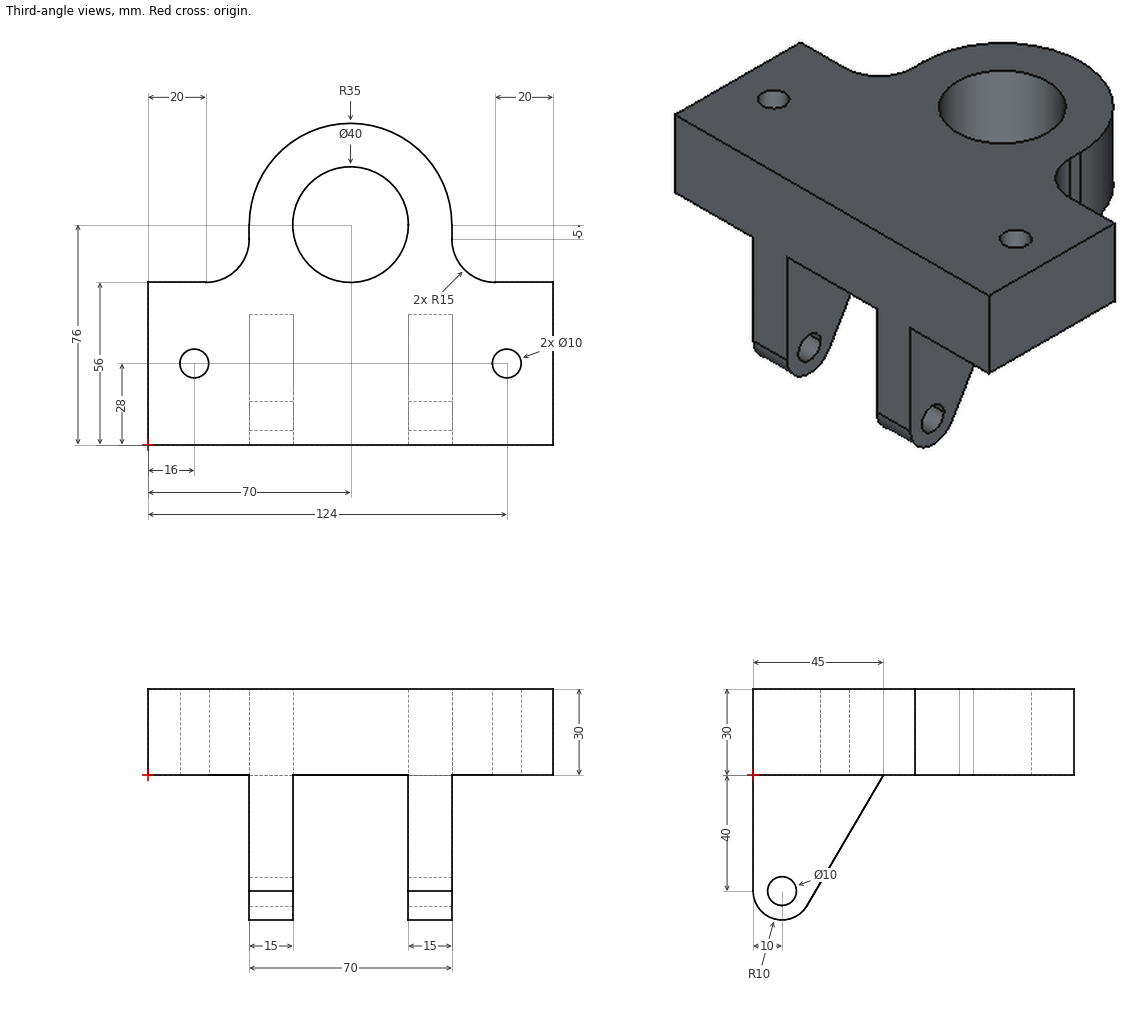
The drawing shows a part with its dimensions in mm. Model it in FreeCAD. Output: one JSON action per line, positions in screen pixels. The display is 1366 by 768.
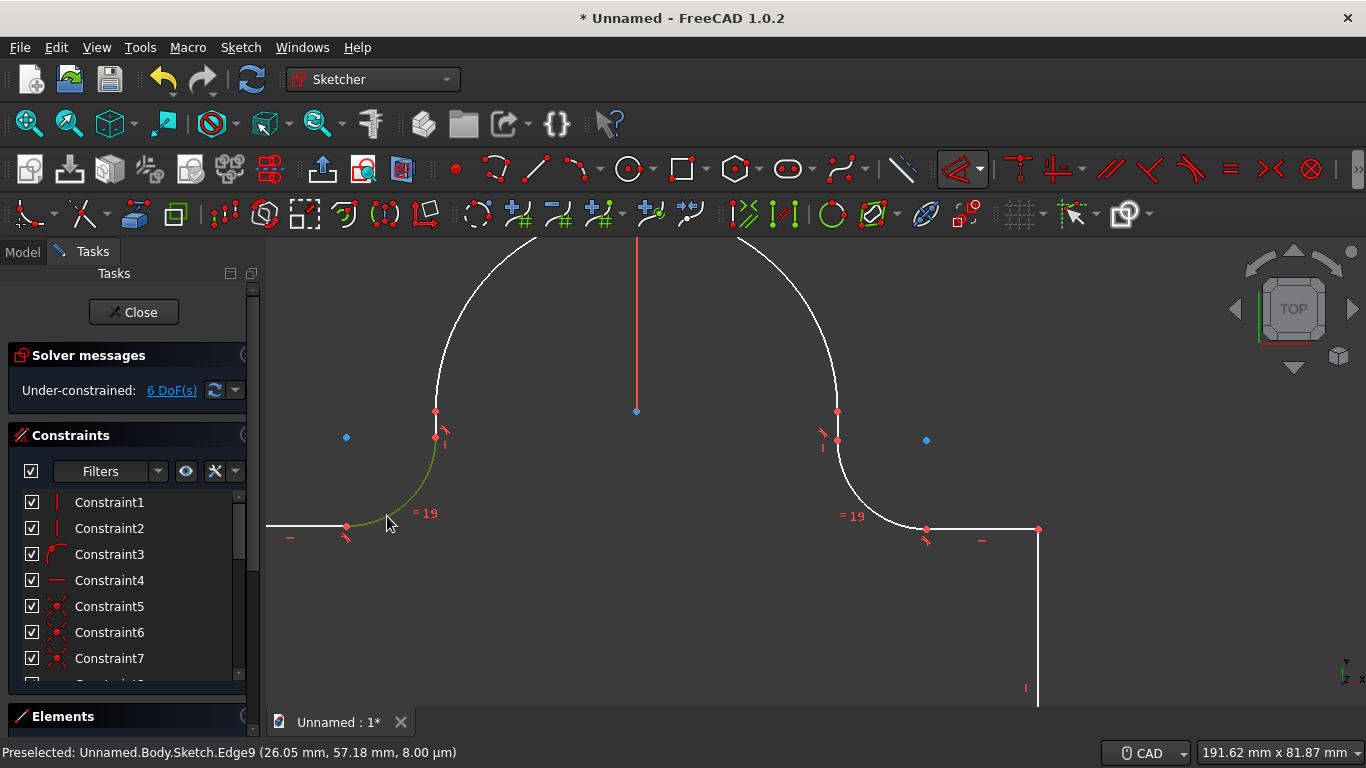
{"action": "left_click", "coordinate": [982, 170]}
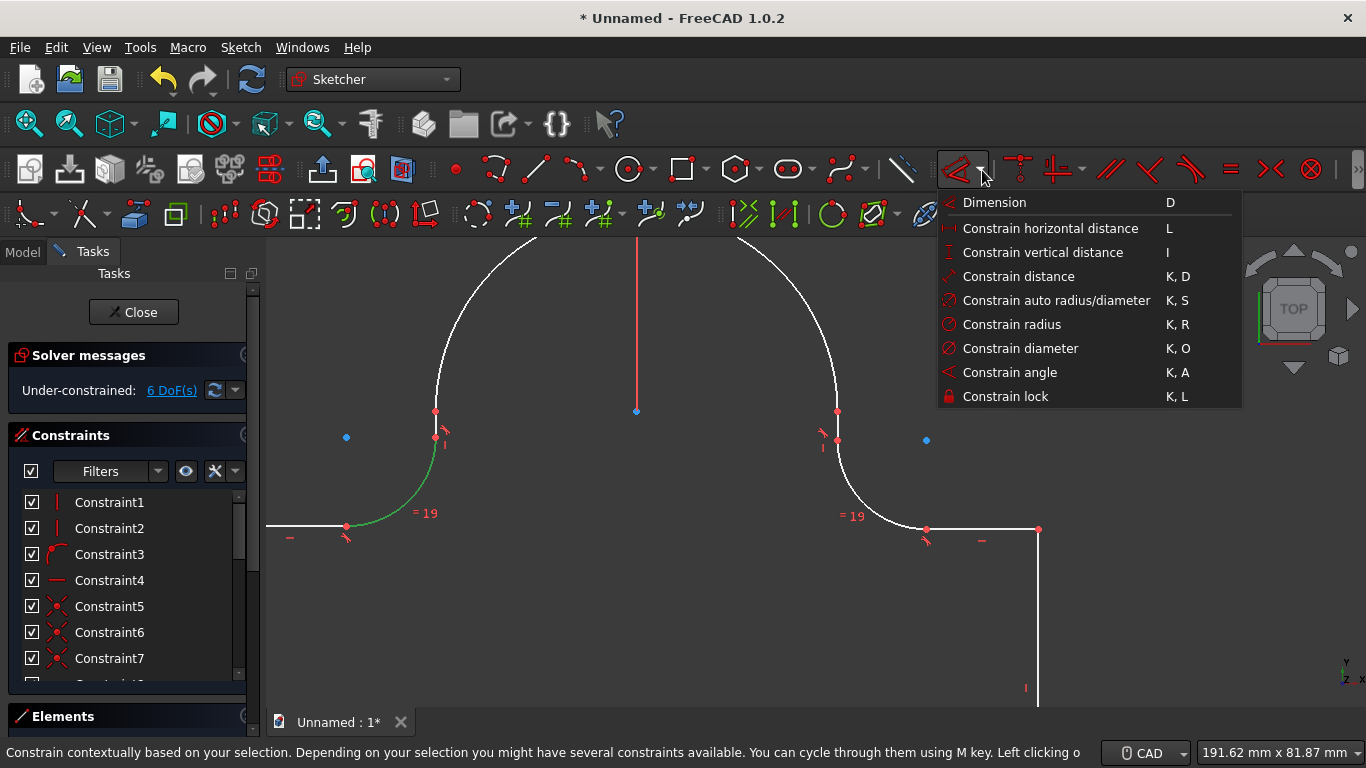
{"action": "left_click", "coordinate": [1090, 324]}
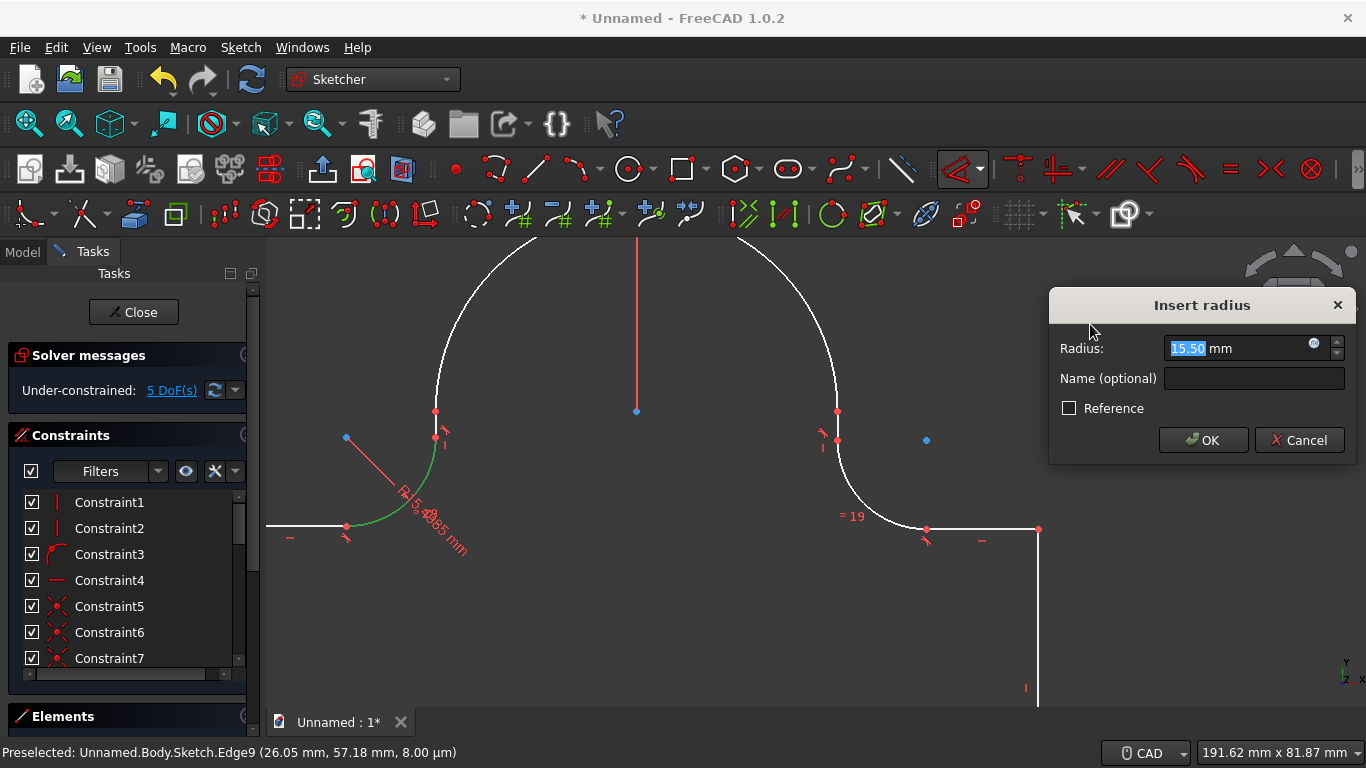
{"action": "type", "text": "15"}
{"action": "key", "text": "Return"}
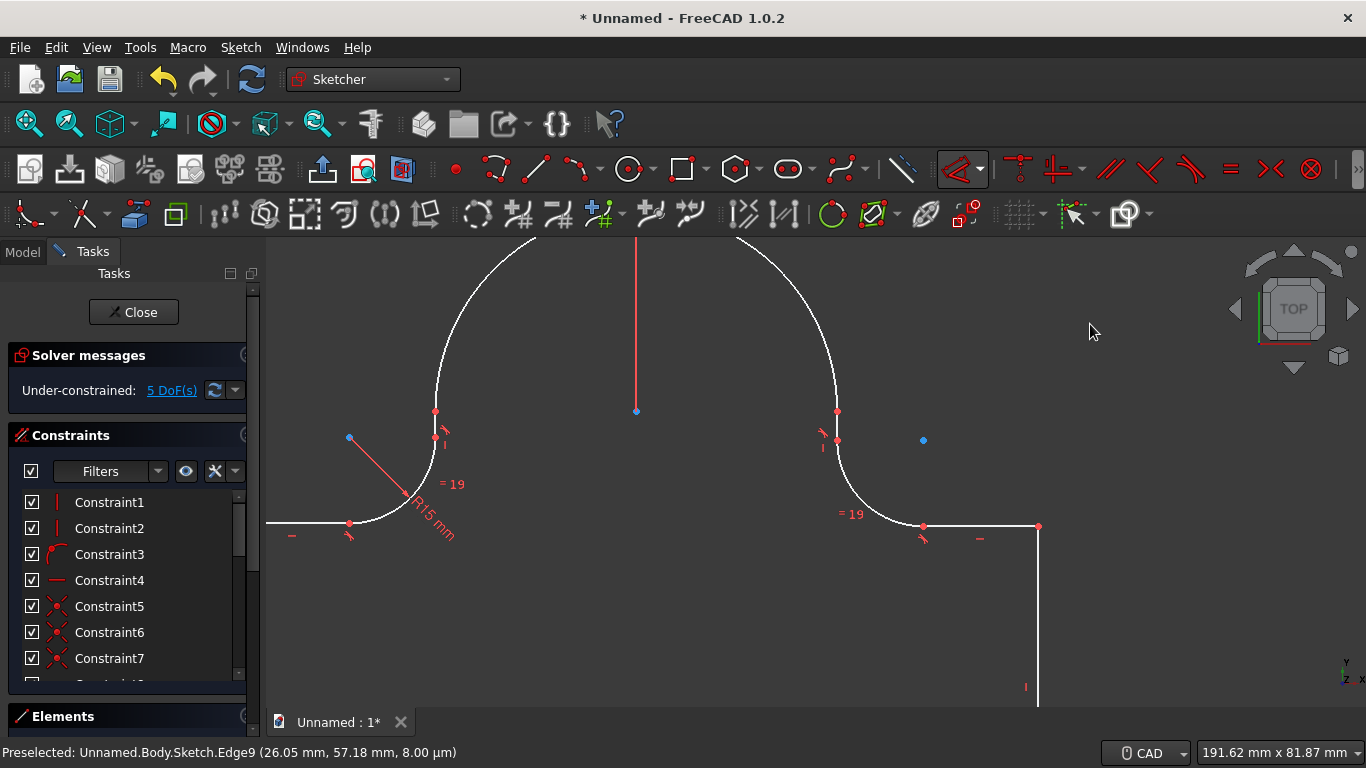
{"action": "scroll", "coordinate": [837, 429], "scroll_direction": "up", "scroll_amount": 2}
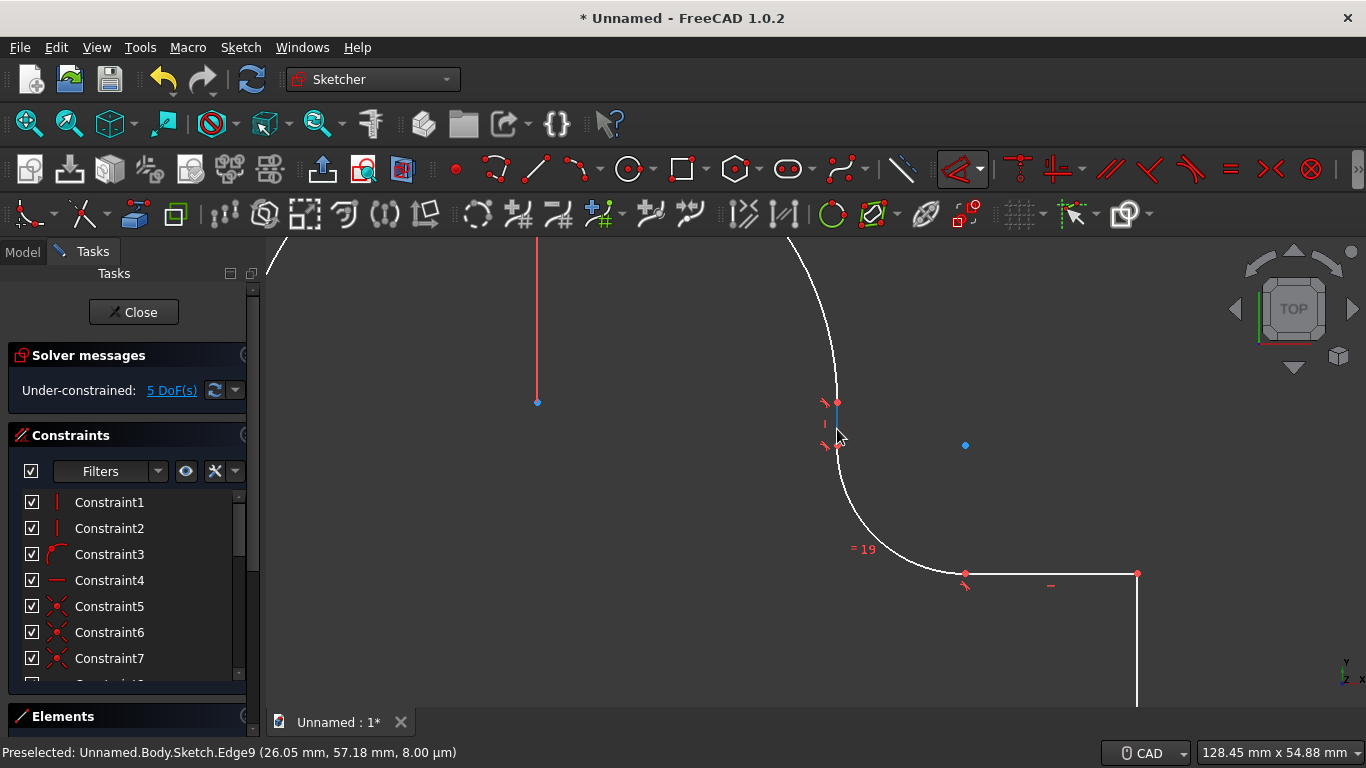
{"action": "left_click", "coordinate": [837, 428]}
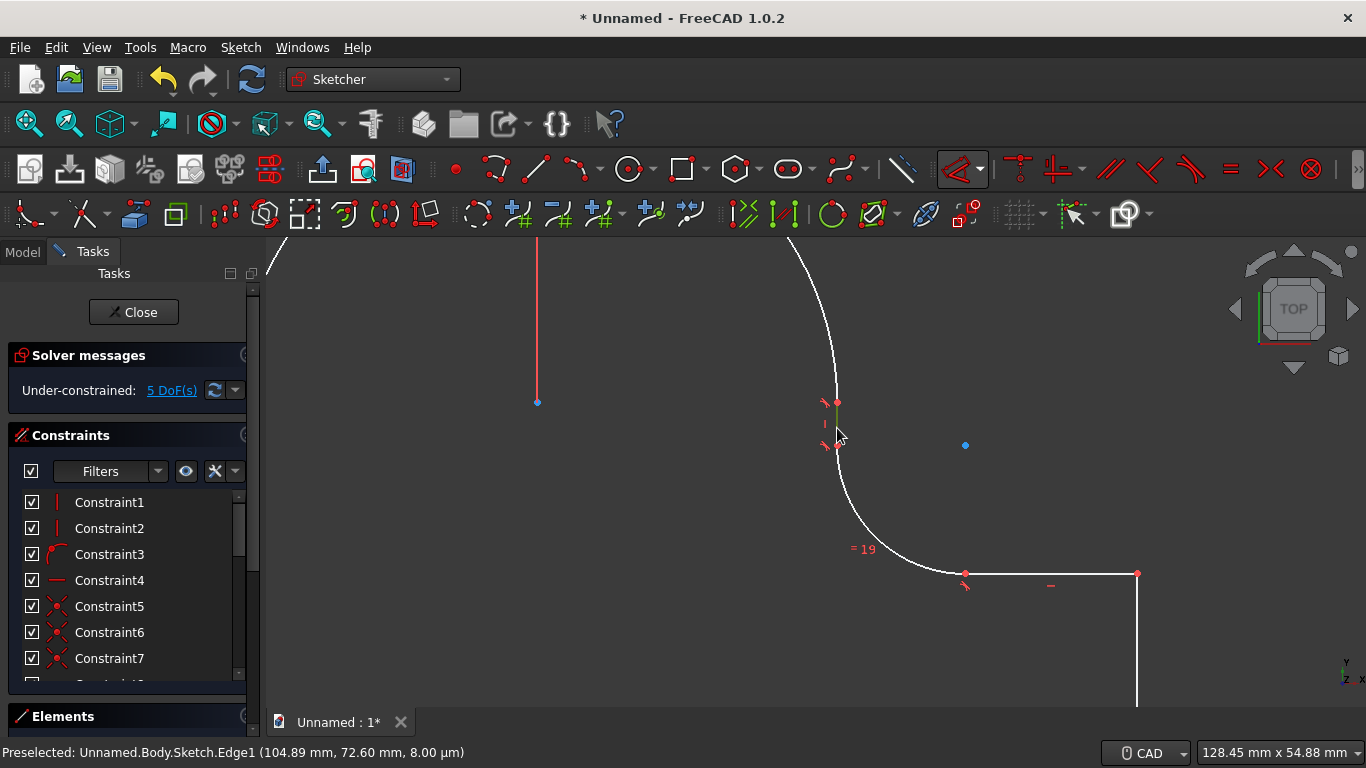
{"action": "left_click", "coordinate": [982, 170]}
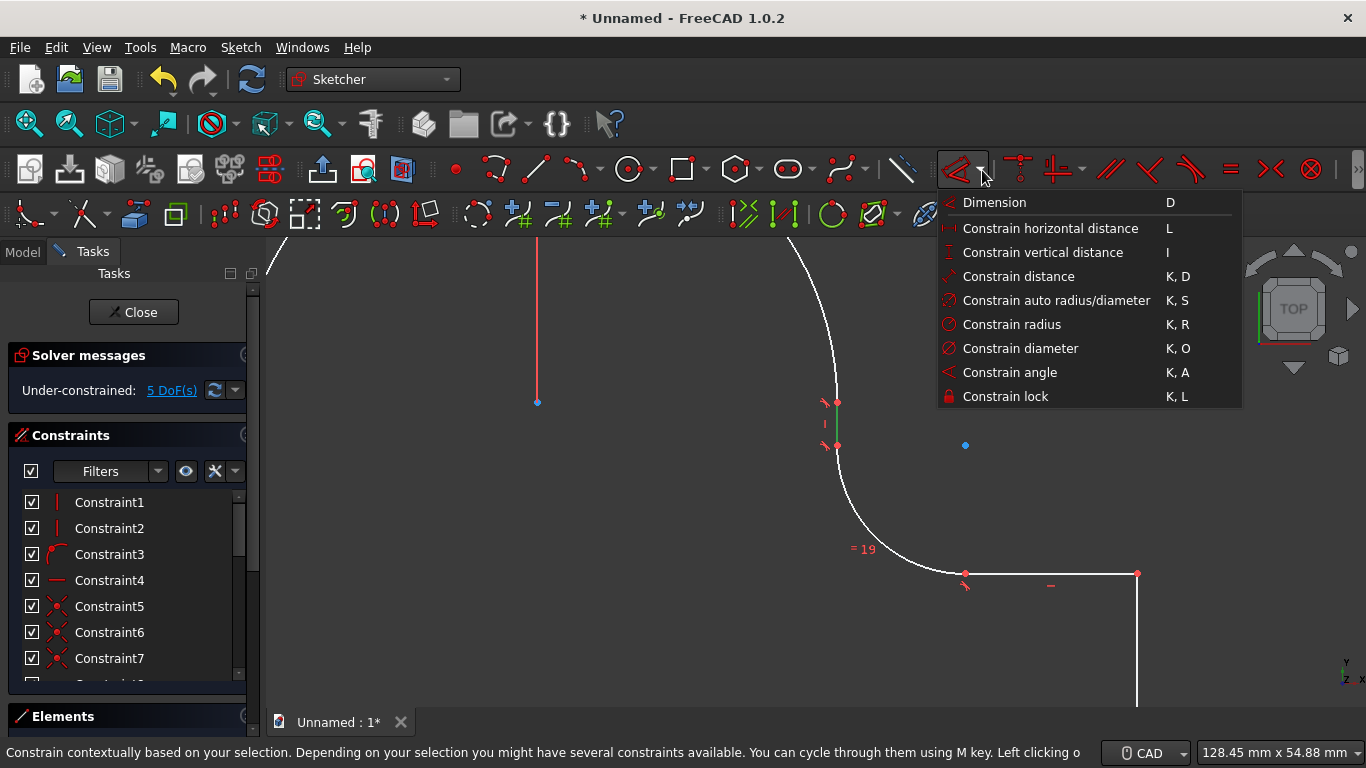
{"action": "left_click", "coordinate": [1090, 252]}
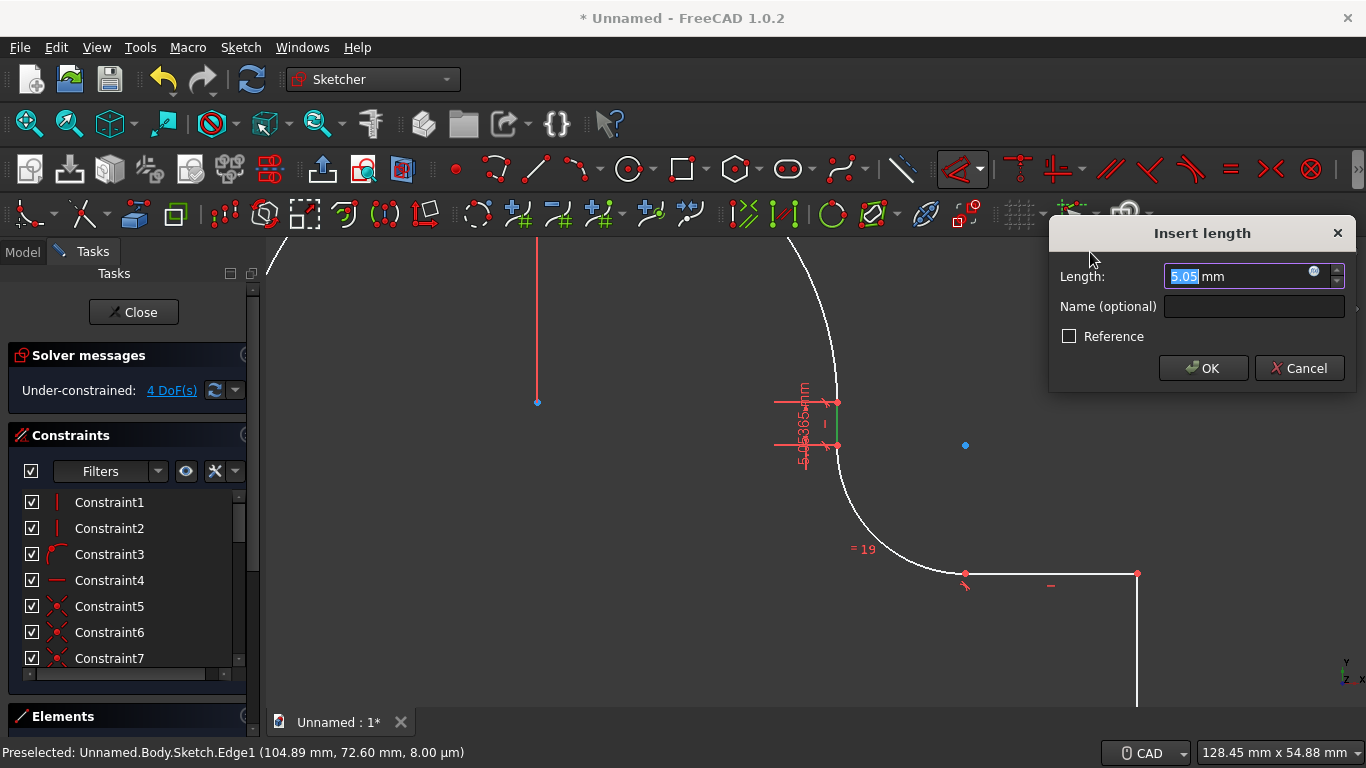
{"action": "type", "text": "5"}
{"action": "key", "text": "Return"}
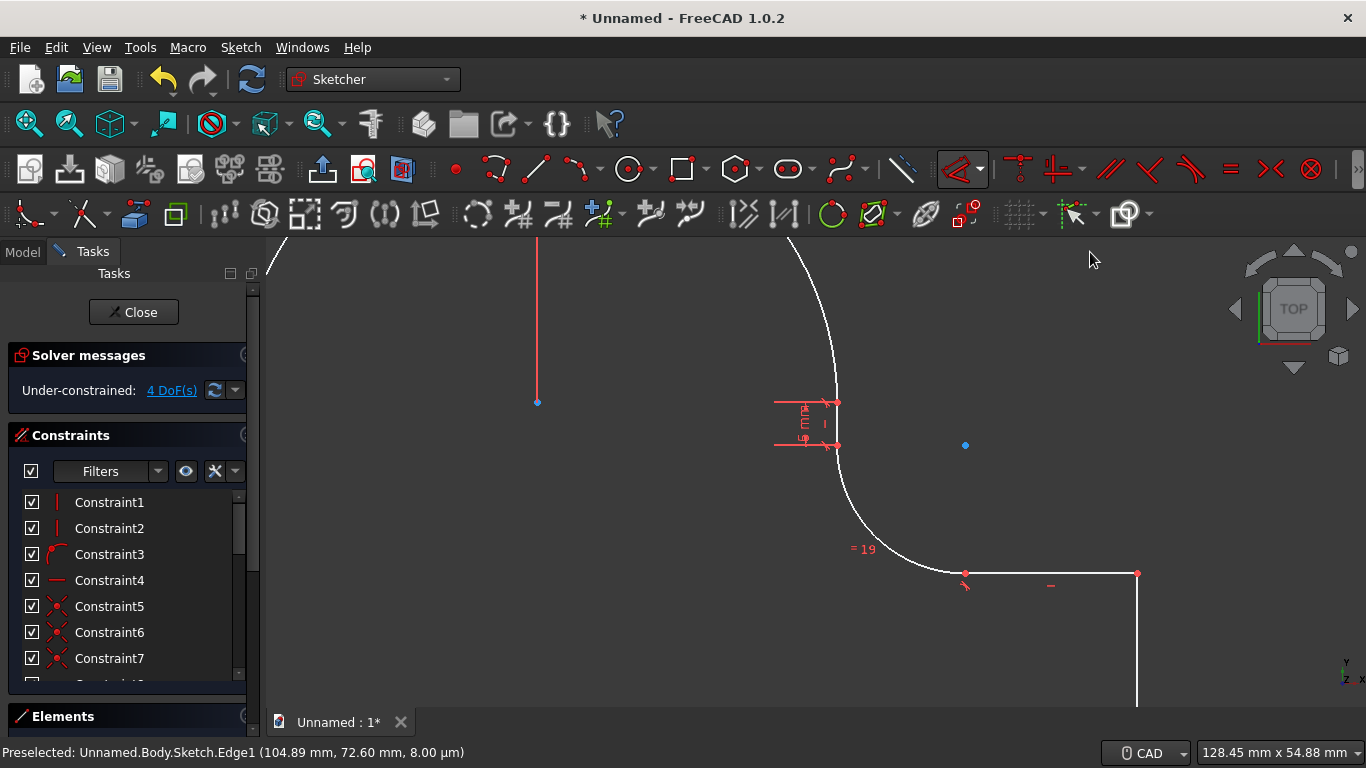
{"action": "scroll", "coordinate": [838, 427], "scroll_direction": "down", "scroll_amount": 6}